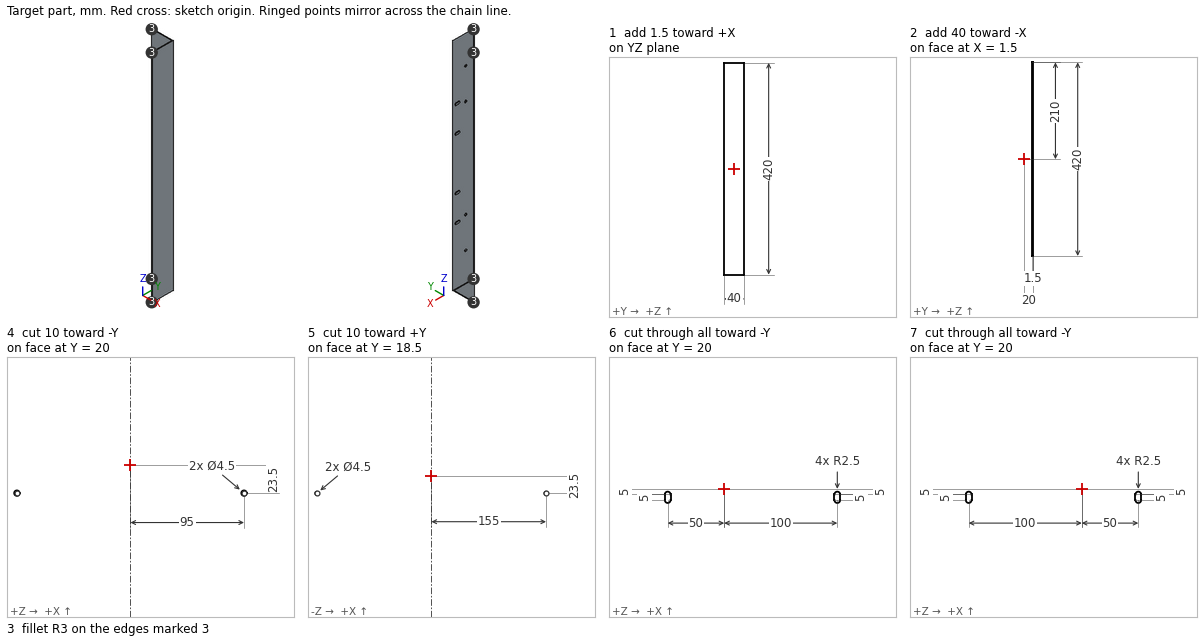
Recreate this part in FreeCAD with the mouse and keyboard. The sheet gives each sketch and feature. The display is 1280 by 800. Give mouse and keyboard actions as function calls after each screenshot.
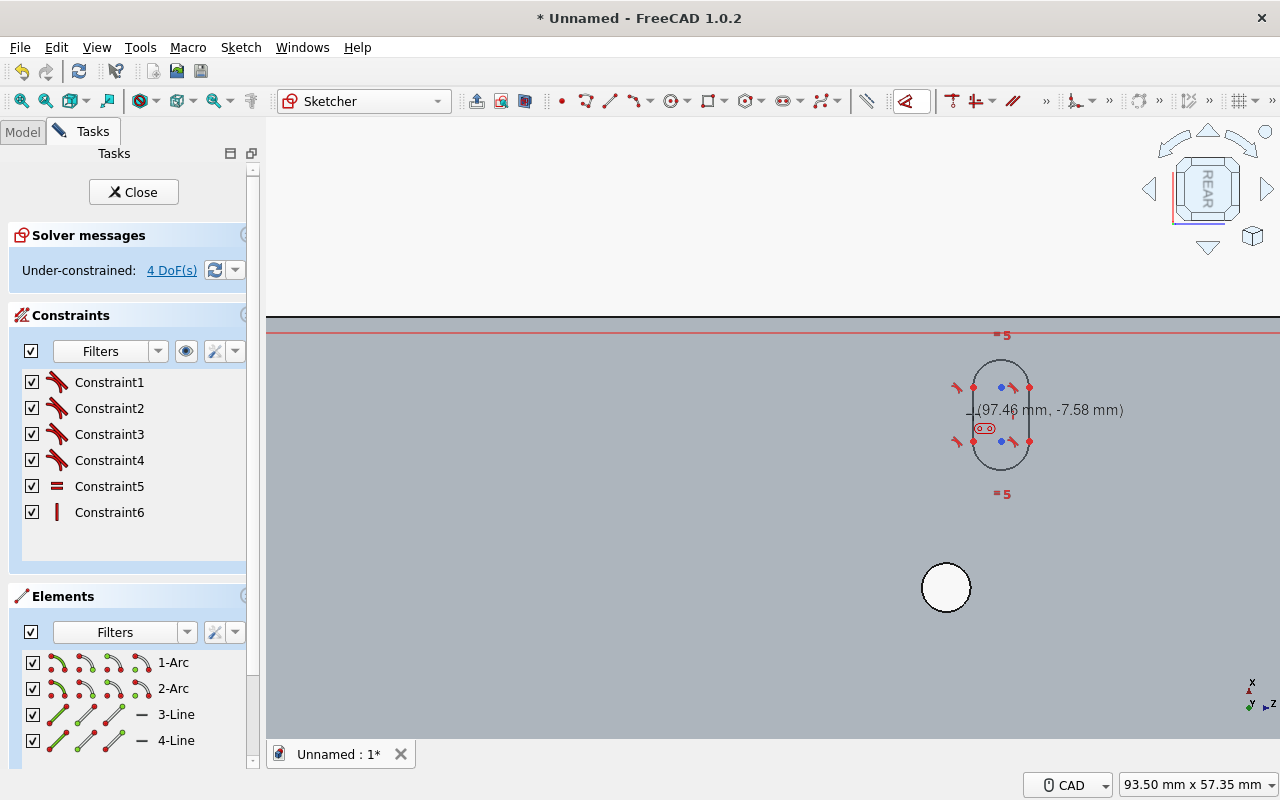
scroll(1006, 444, down, 5)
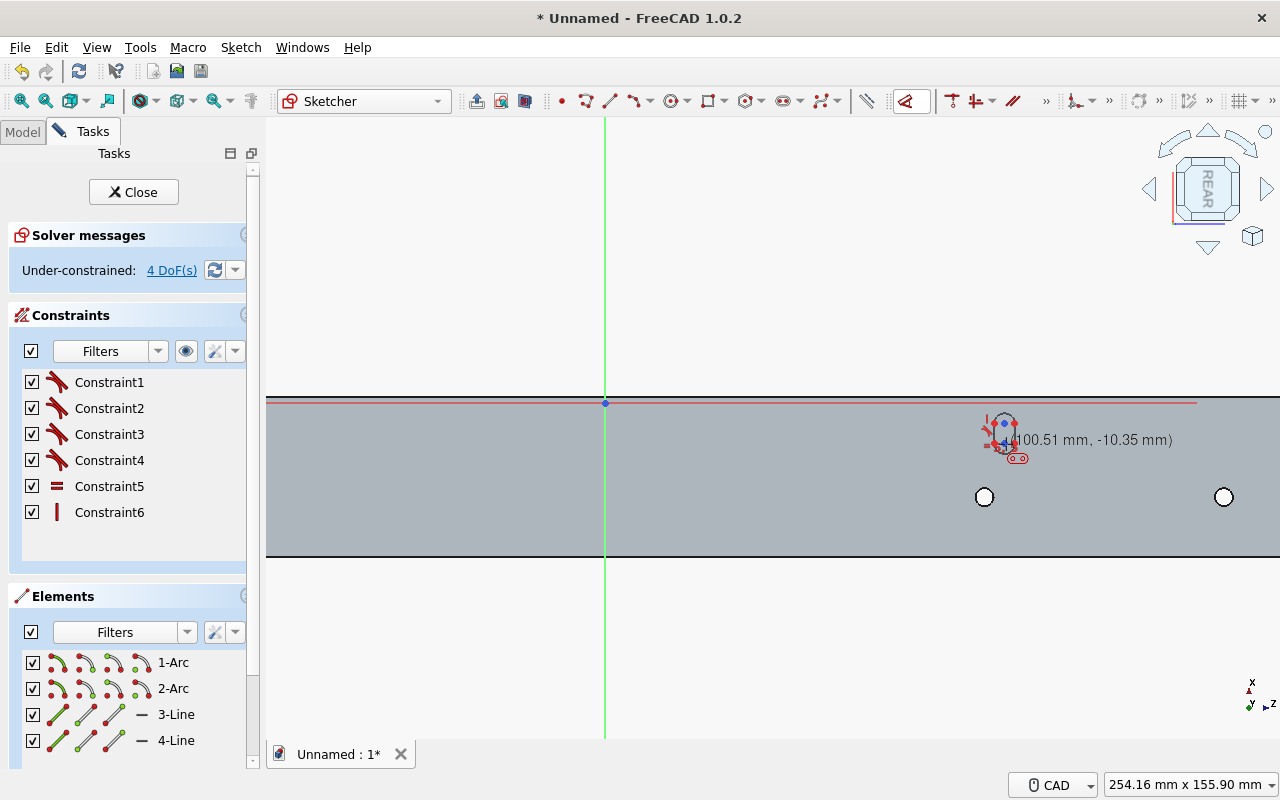
scroll(406, 443, up, 5)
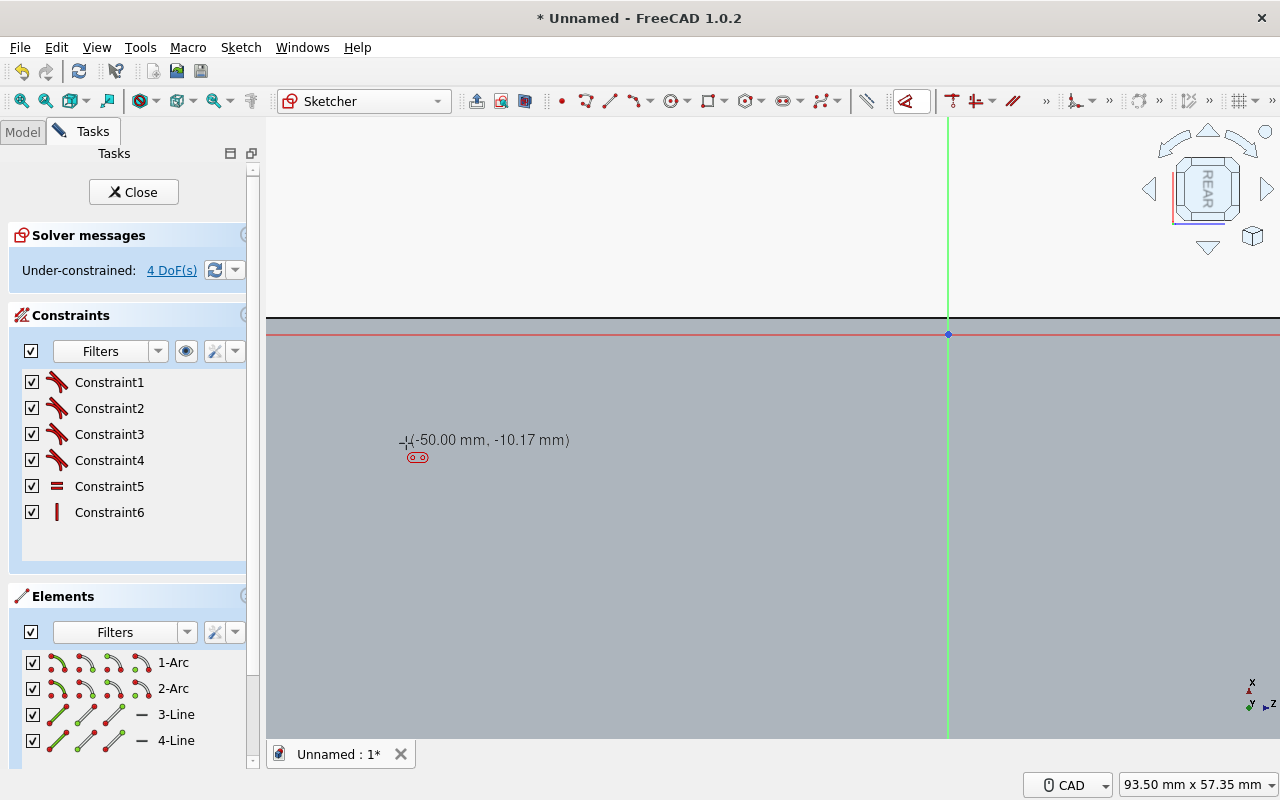
click(406, 443)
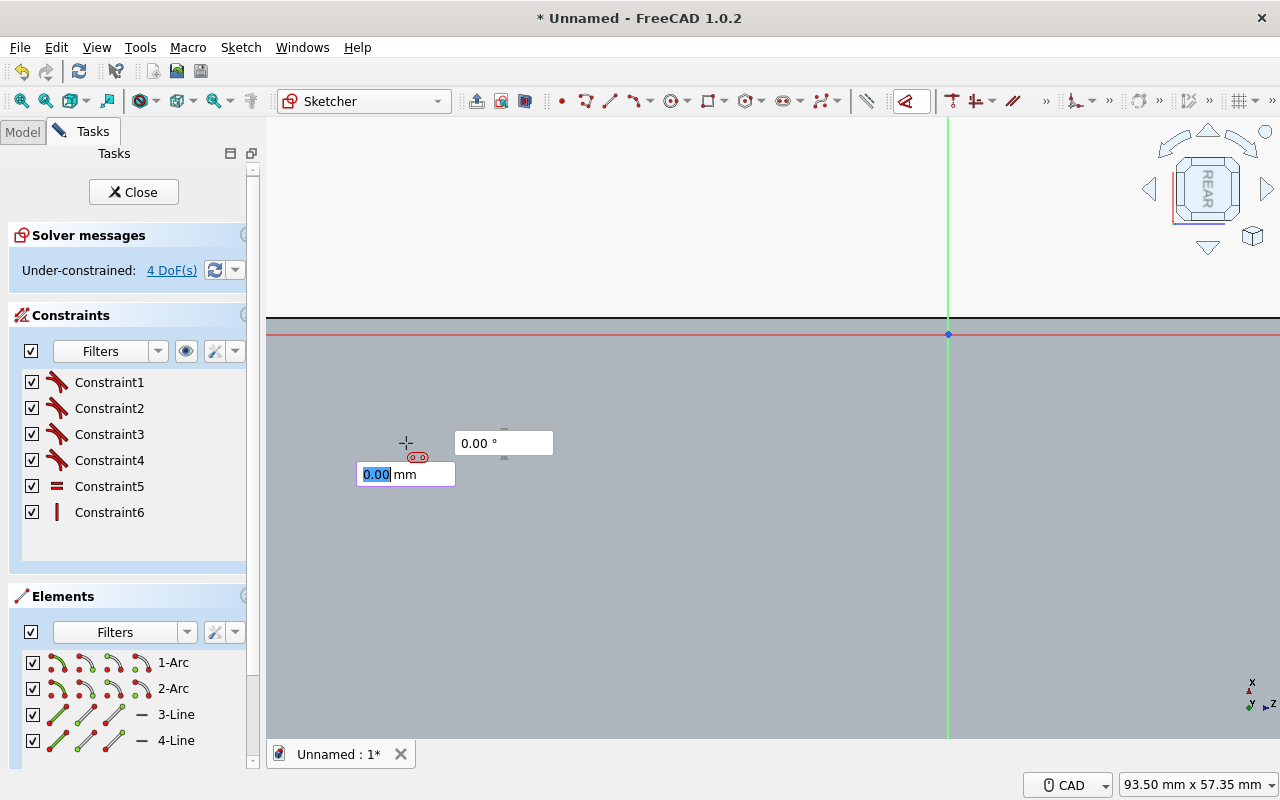
click(406, 389)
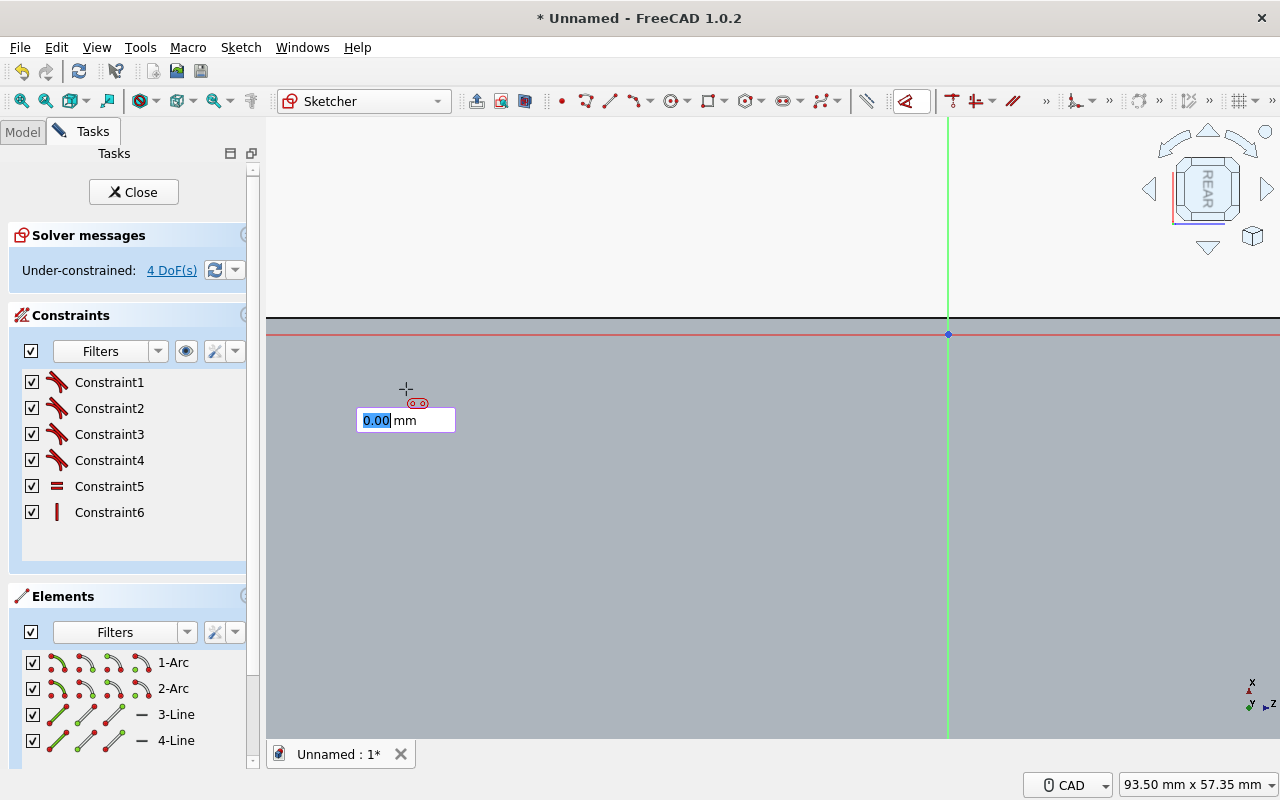
click(433, 416)
key(Escape)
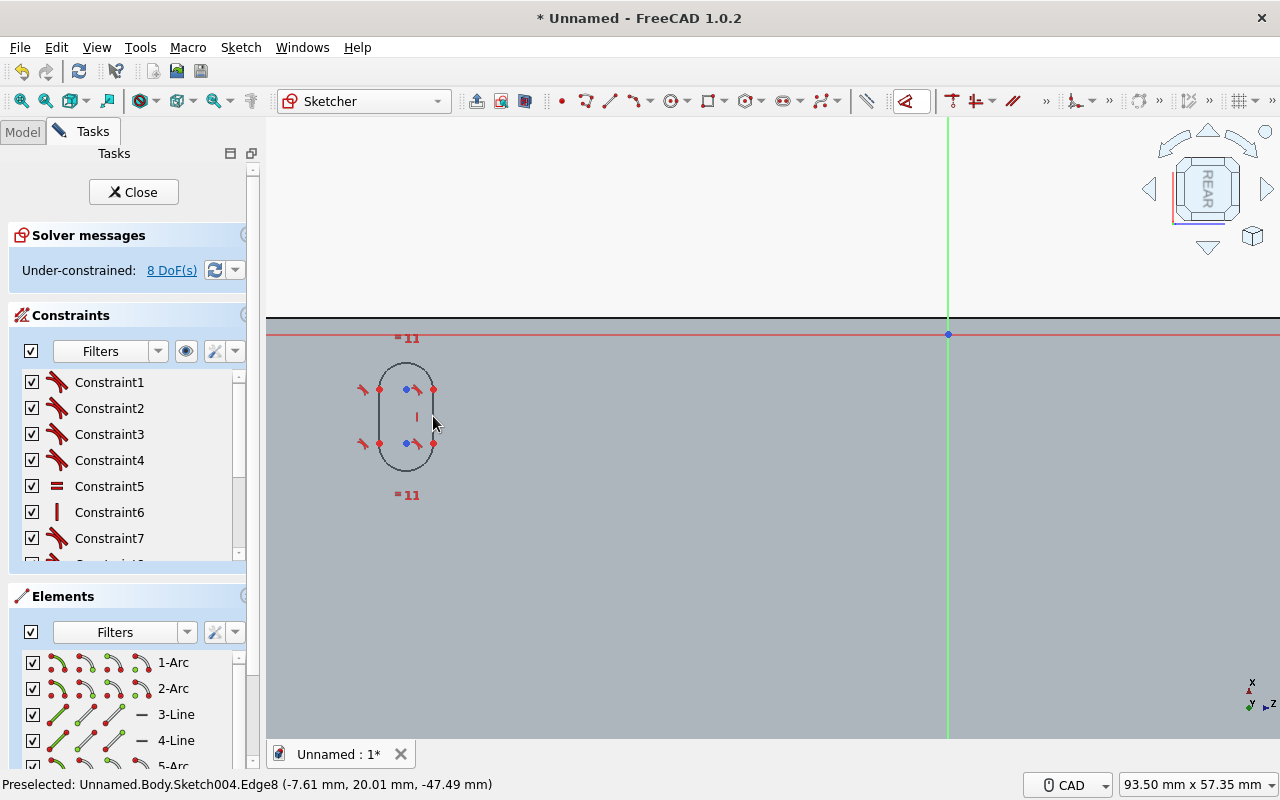
scroll(405, 443, down, 5)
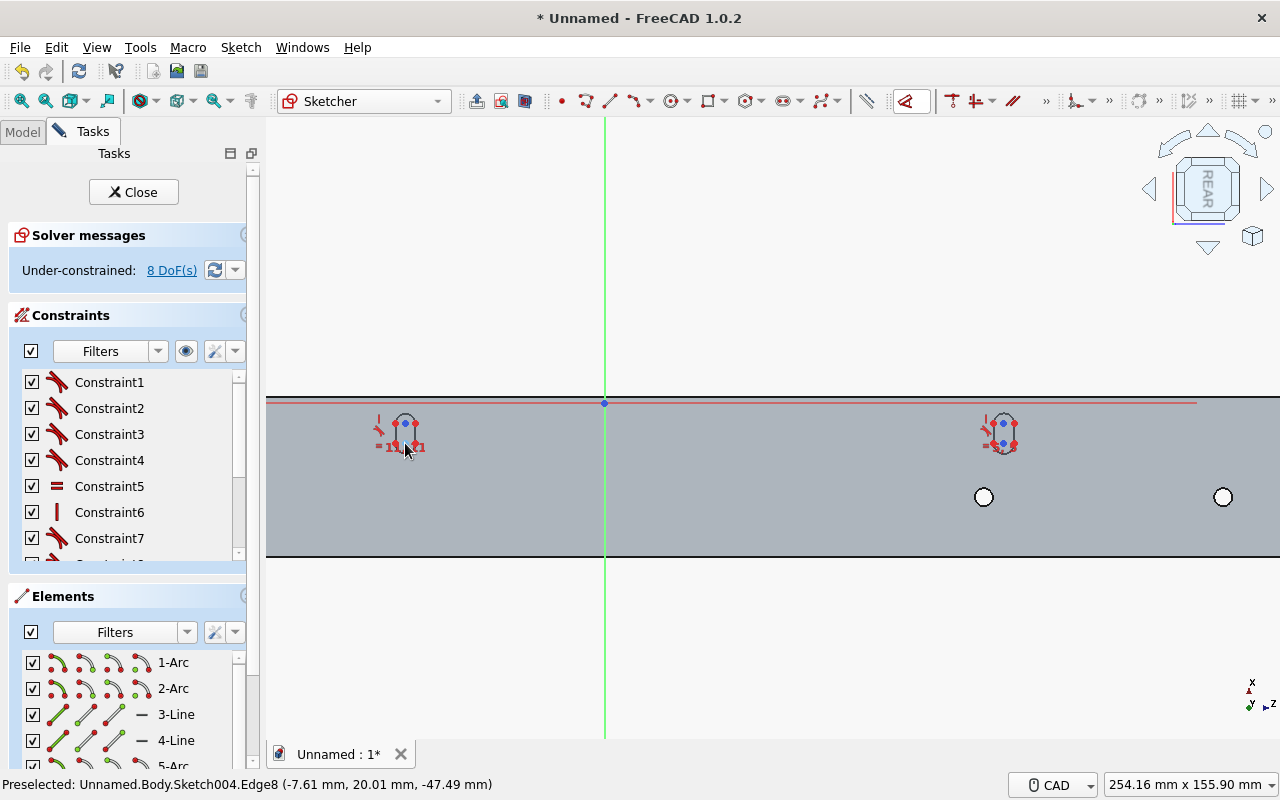
scroll(998, 452, up, 2)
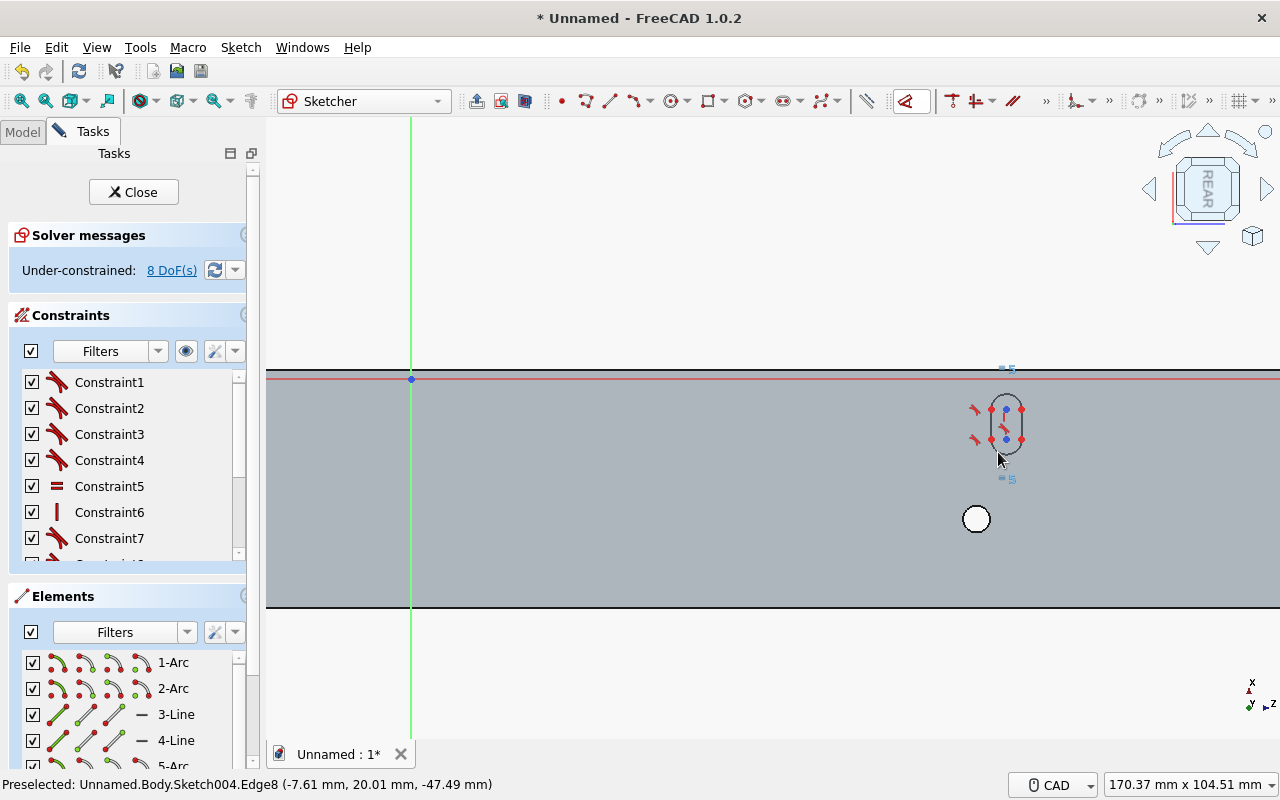
click(998, 452)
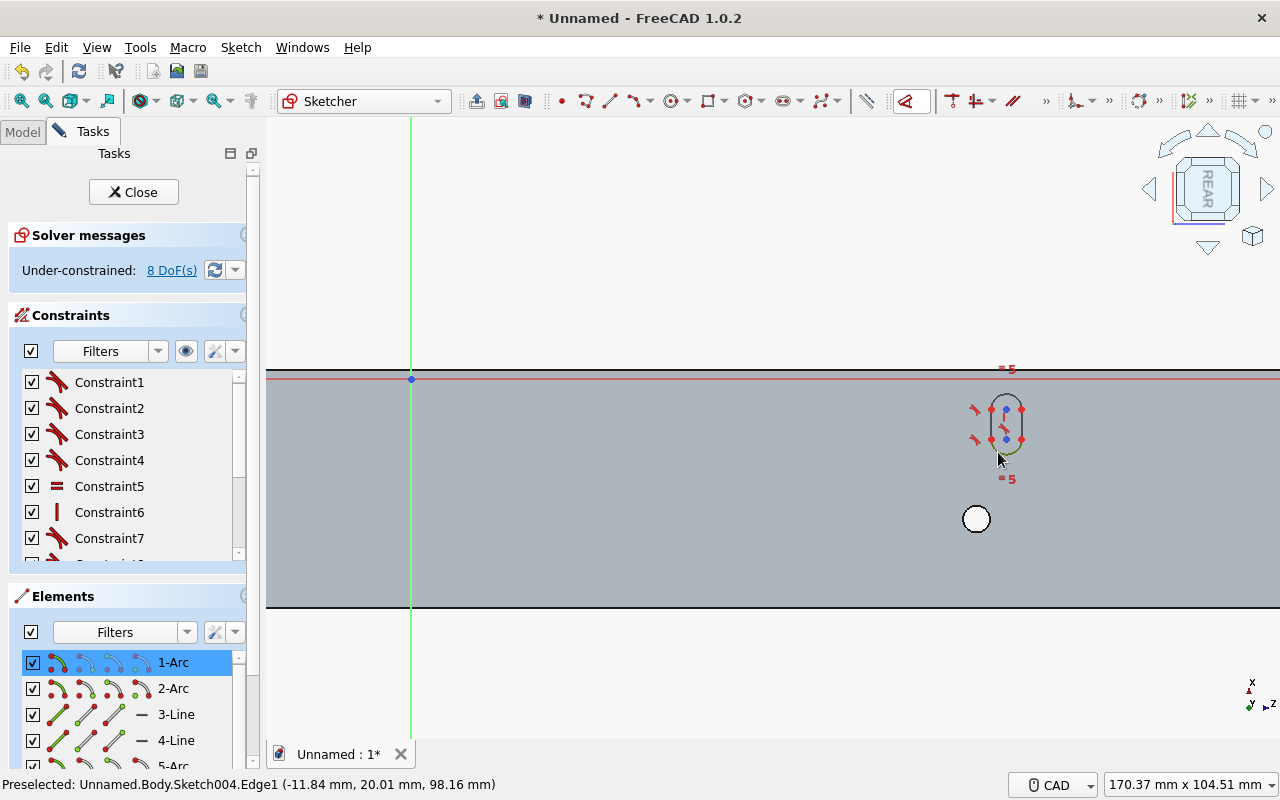
scroll(998, 451, down, 2)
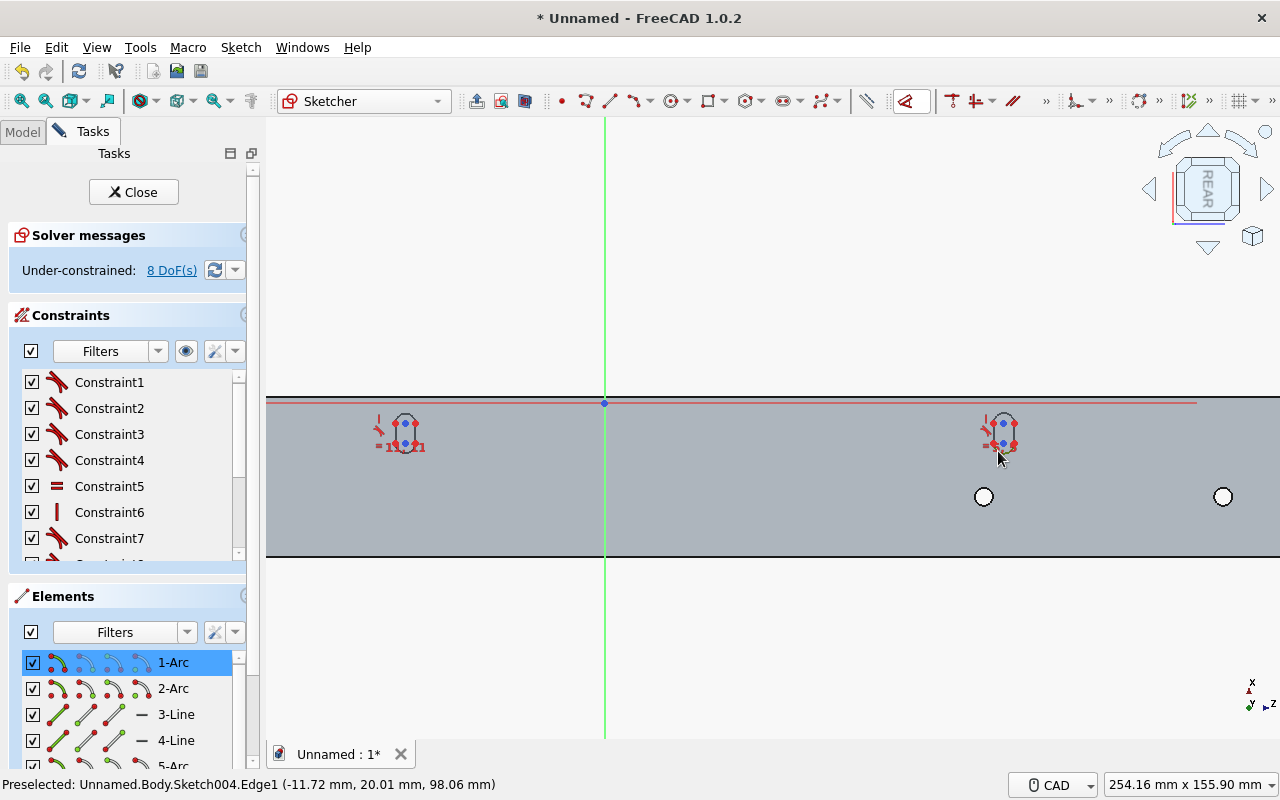
scroll(400, 451, up, 3)